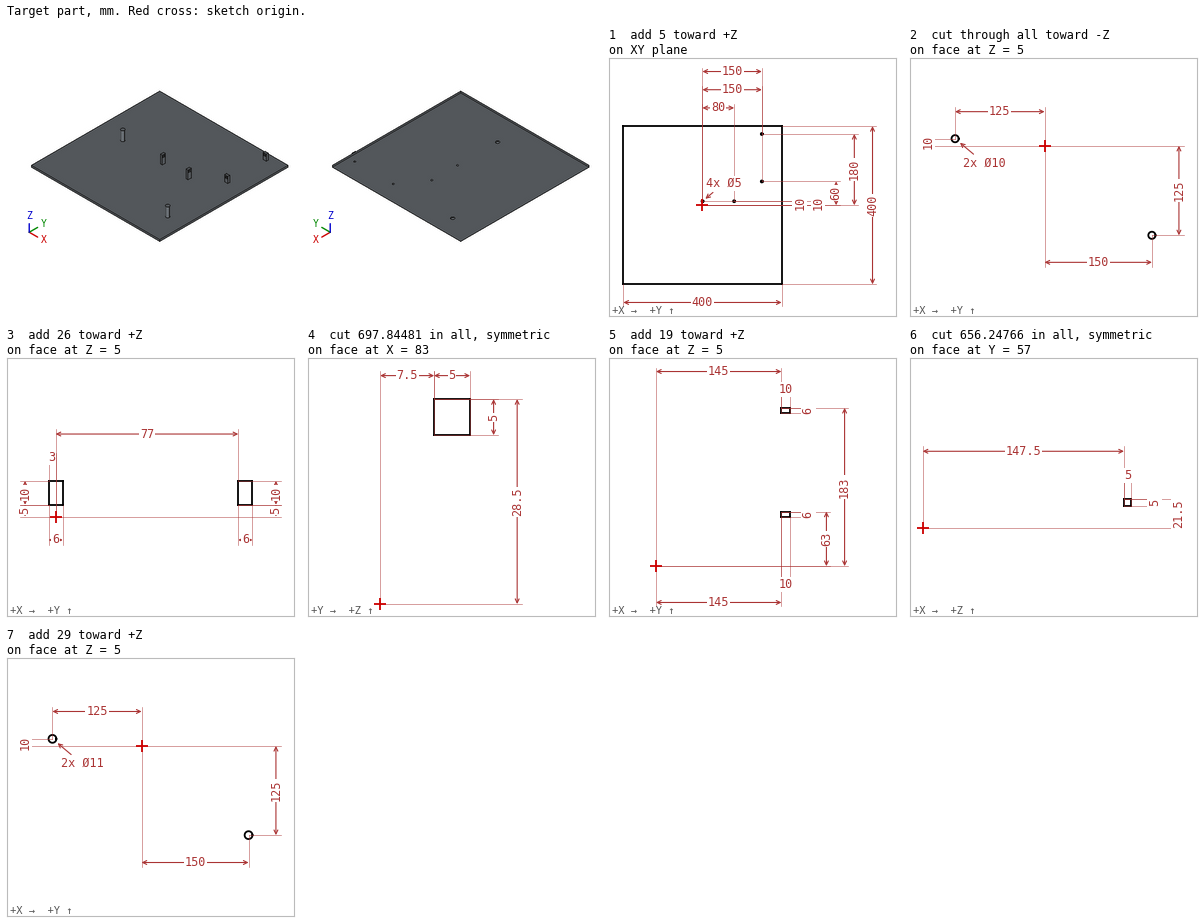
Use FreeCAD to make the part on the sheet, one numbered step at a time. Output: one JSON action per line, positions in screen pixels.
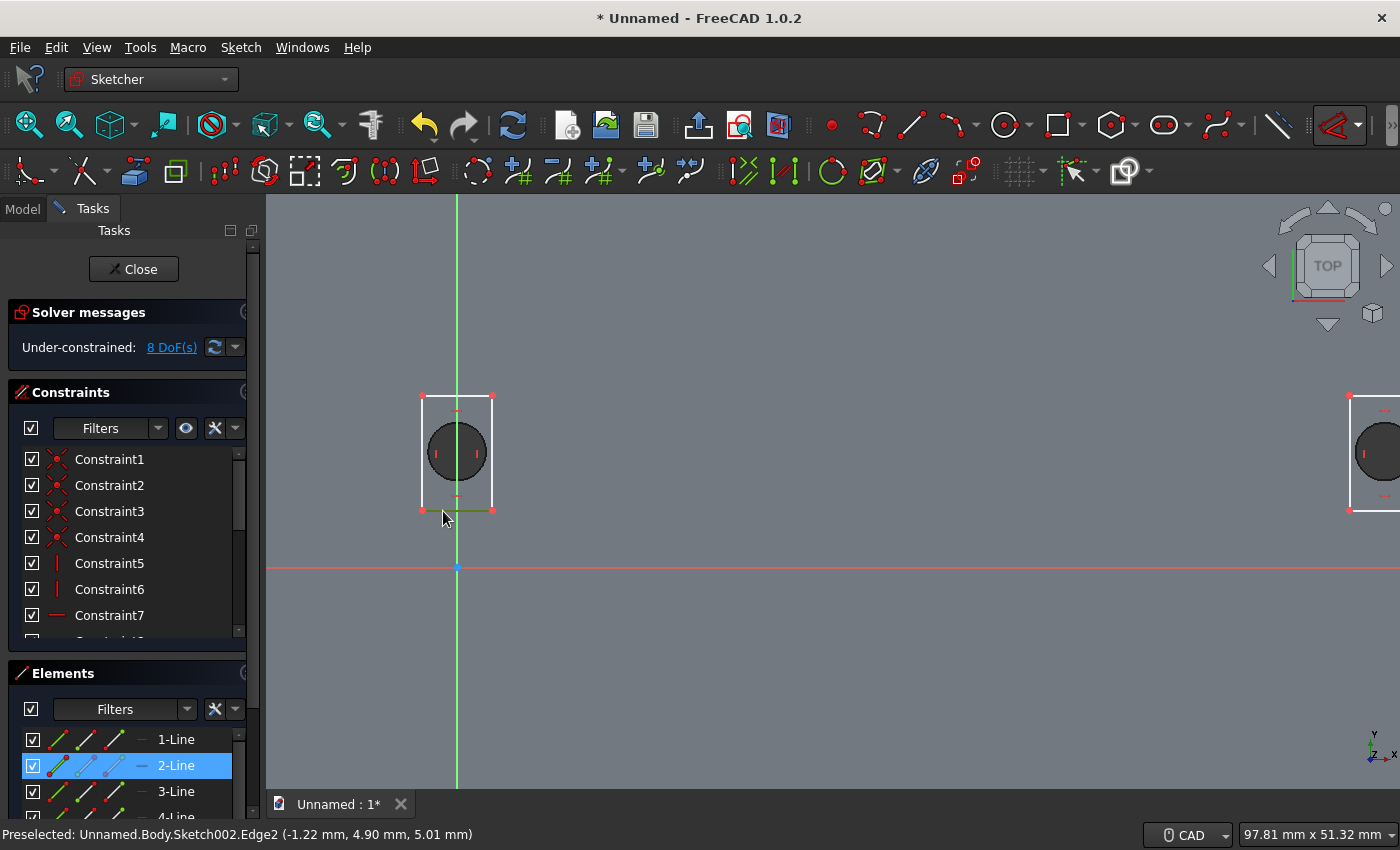
{"action": "key", "text": "l"}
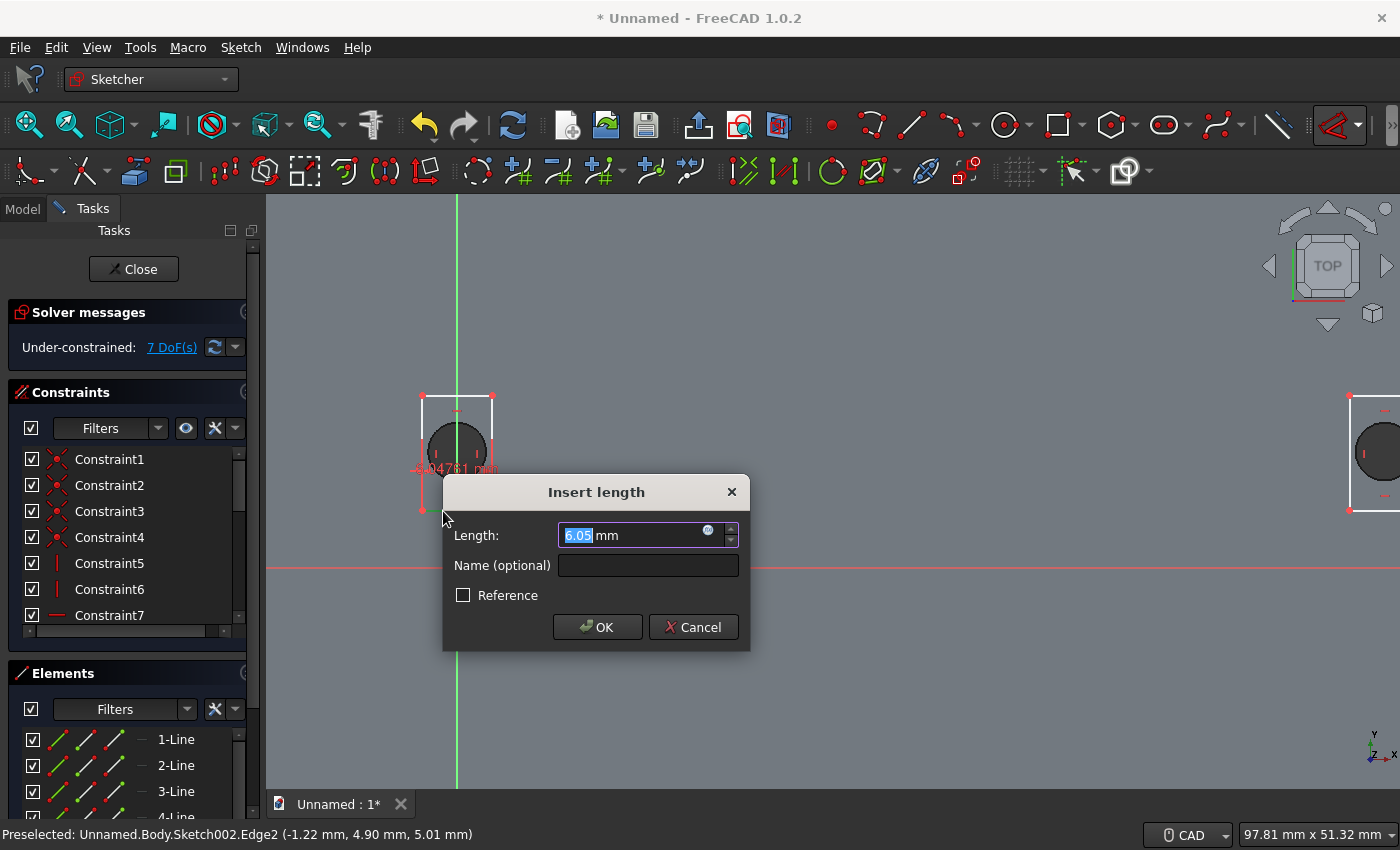
{"action": "type", "text": "6"}
{"action": "key", "text": "Return"}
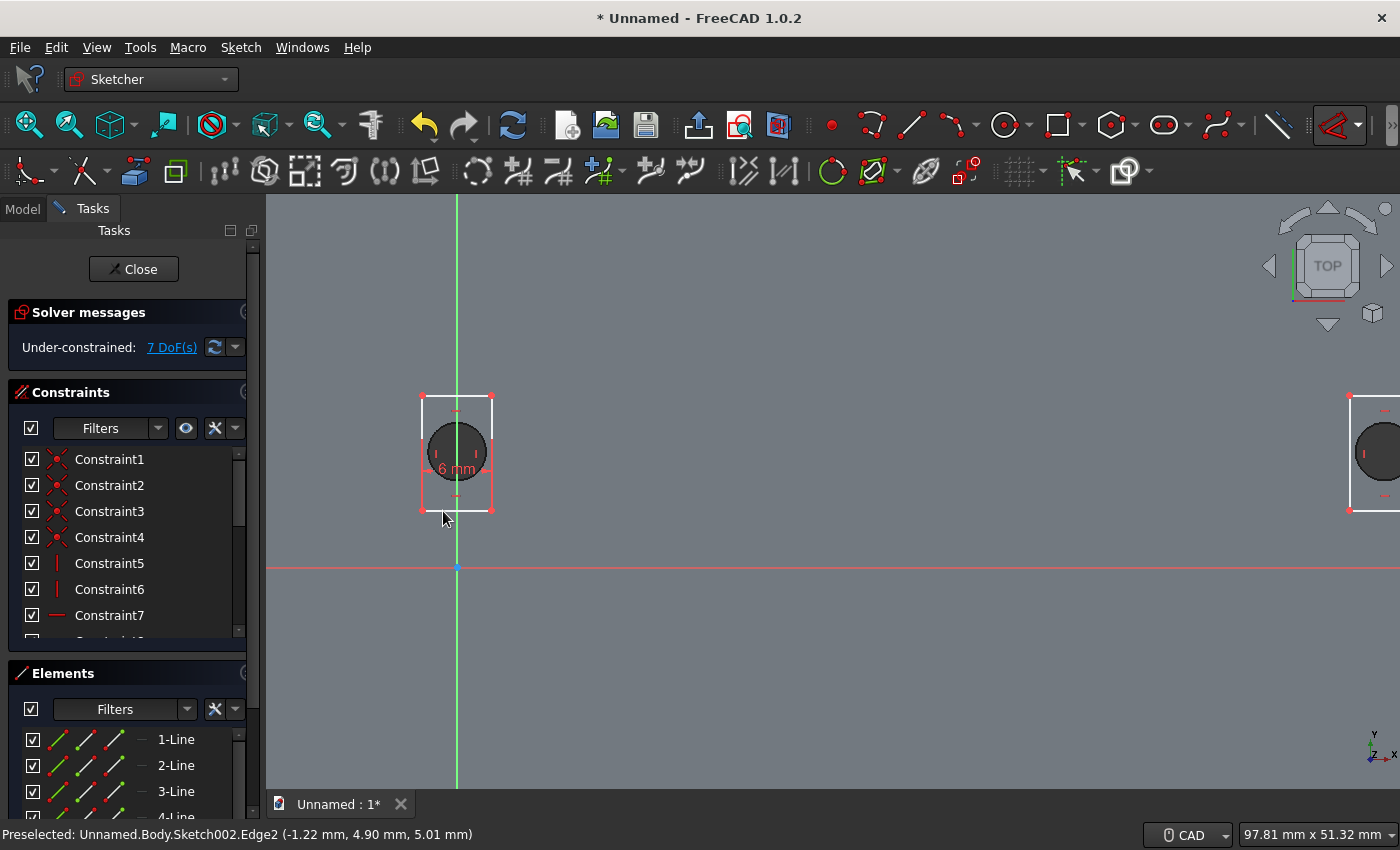
{"action": "scroll", "coordinate": [447, 514], "scroll_direction": "down", "scroll_amount": 2}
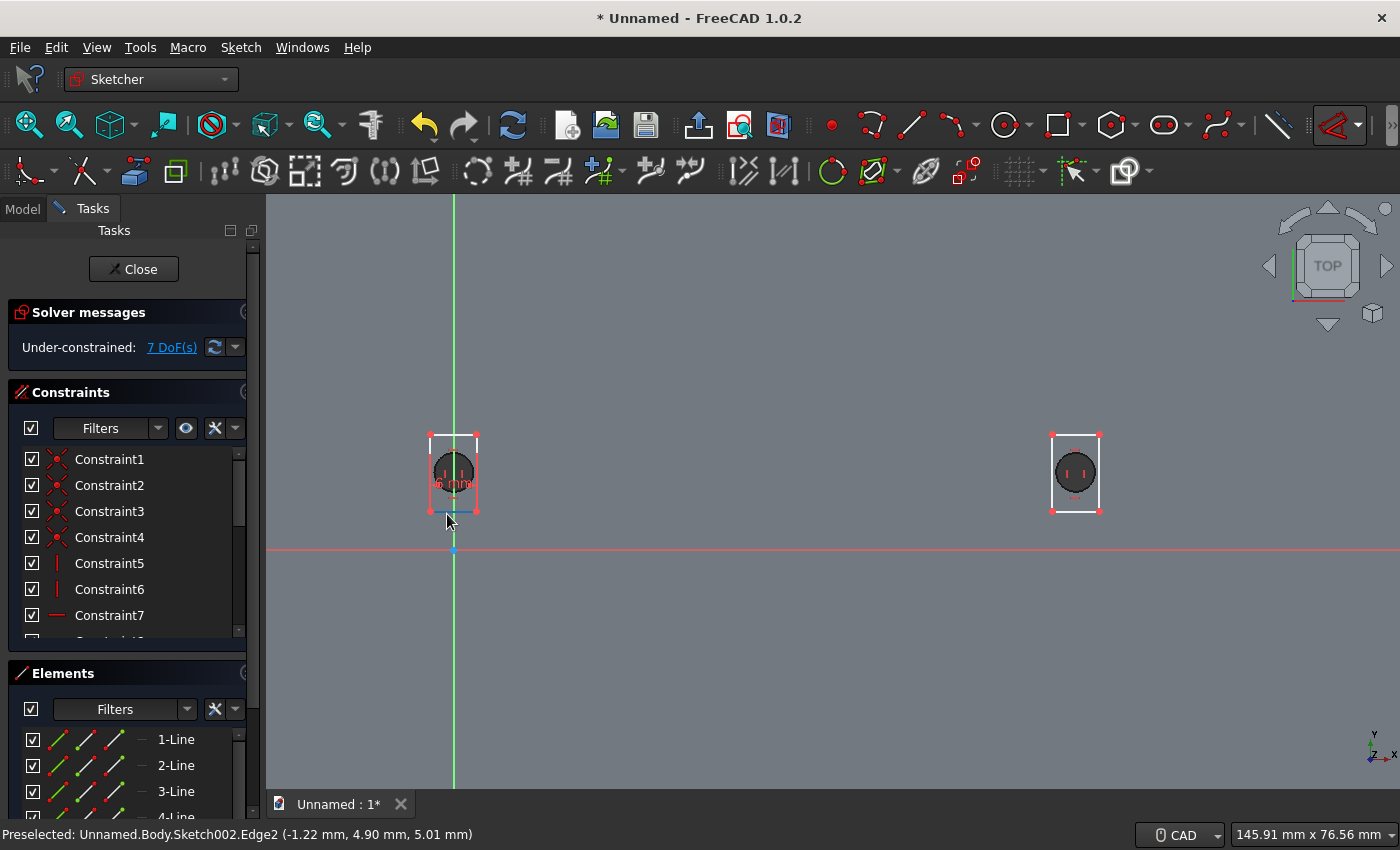
{"action": "left_click", "coordinate": [1066, 512]}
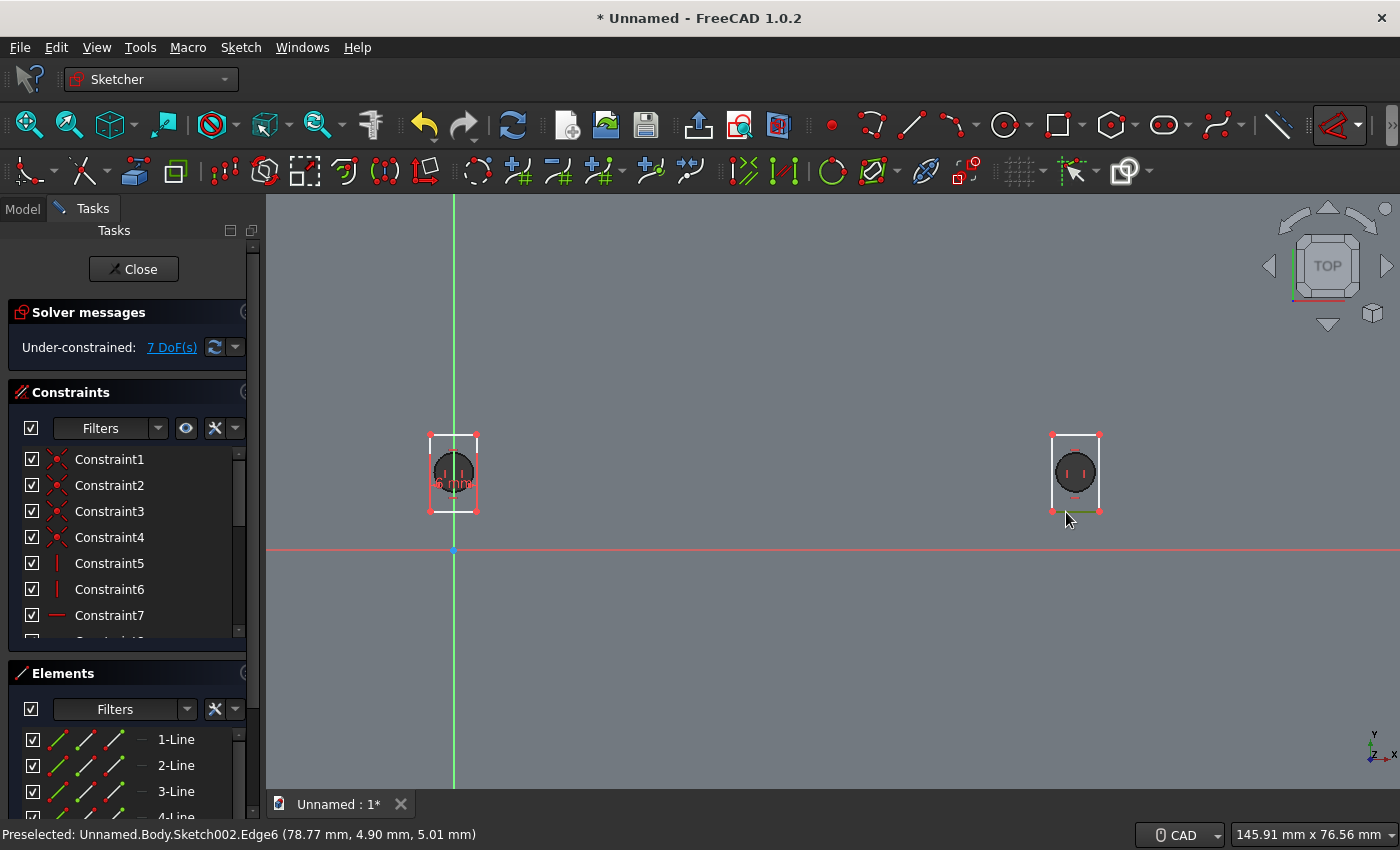
{"action": "key", "text": "l"}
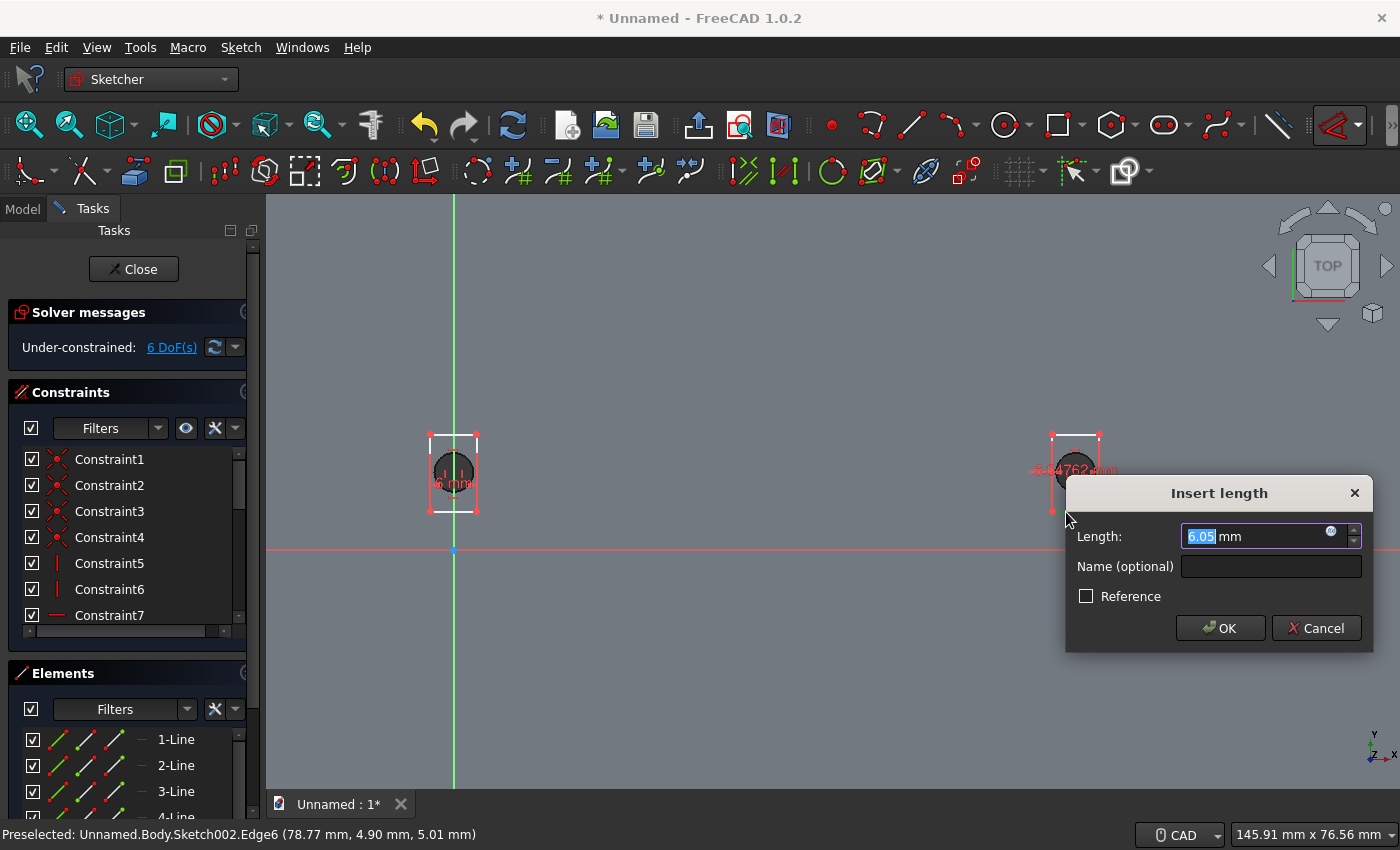
{"action": "type", "text": "6"}
{"action": "key", "text": "Return"}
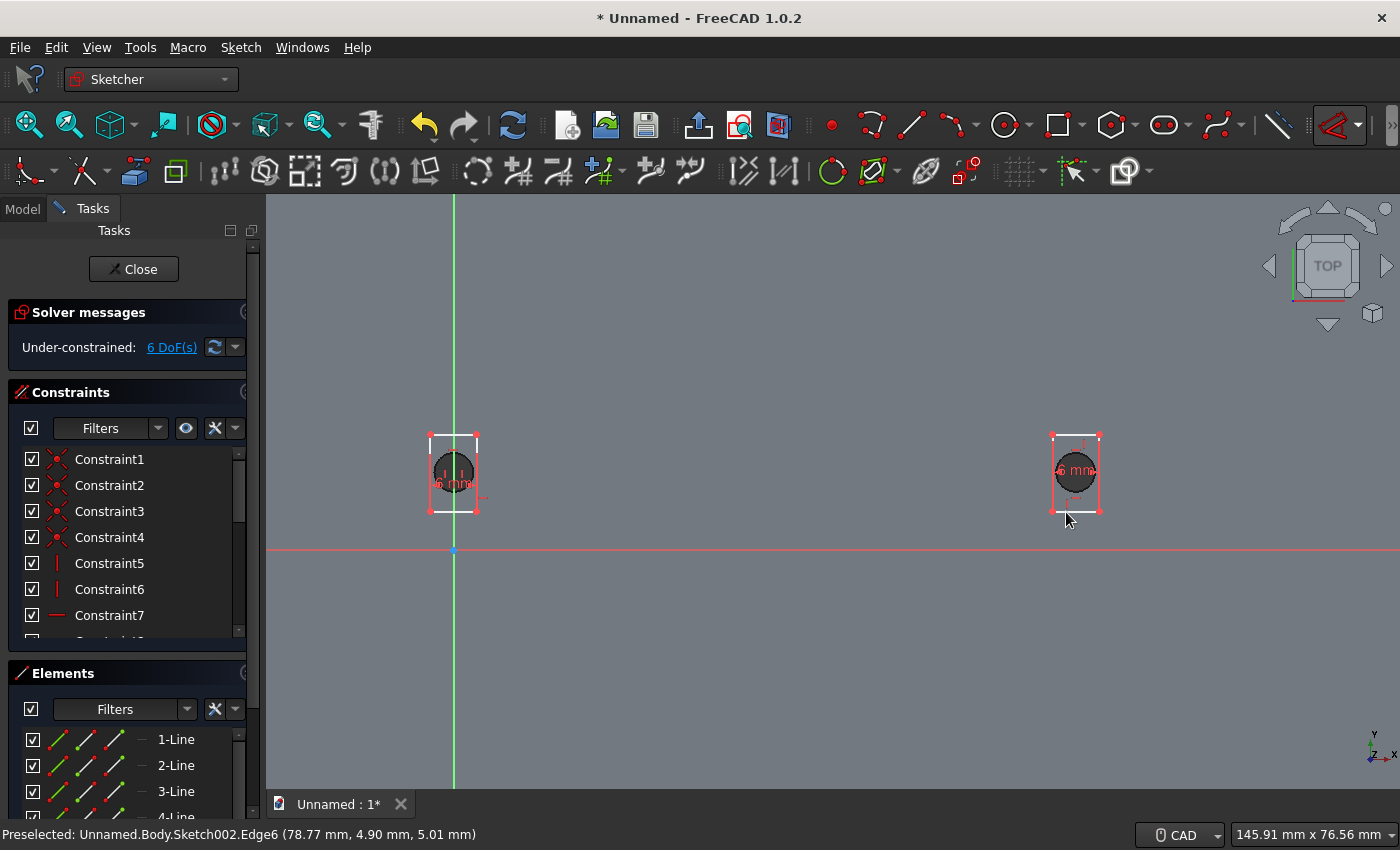
{"action": "left_click", "coordinate": [430, 458]}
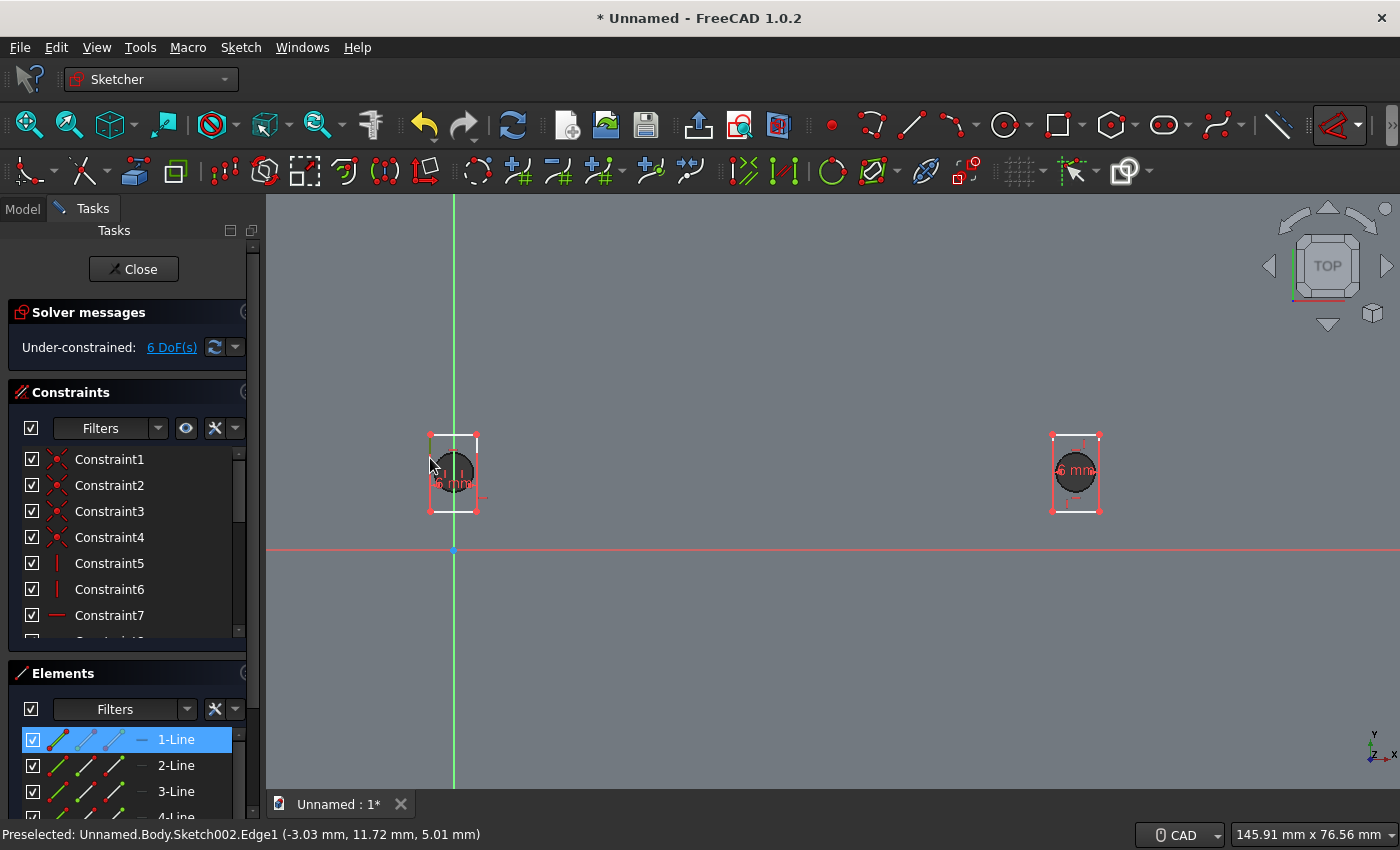
{"action": "key", "text": "i"}